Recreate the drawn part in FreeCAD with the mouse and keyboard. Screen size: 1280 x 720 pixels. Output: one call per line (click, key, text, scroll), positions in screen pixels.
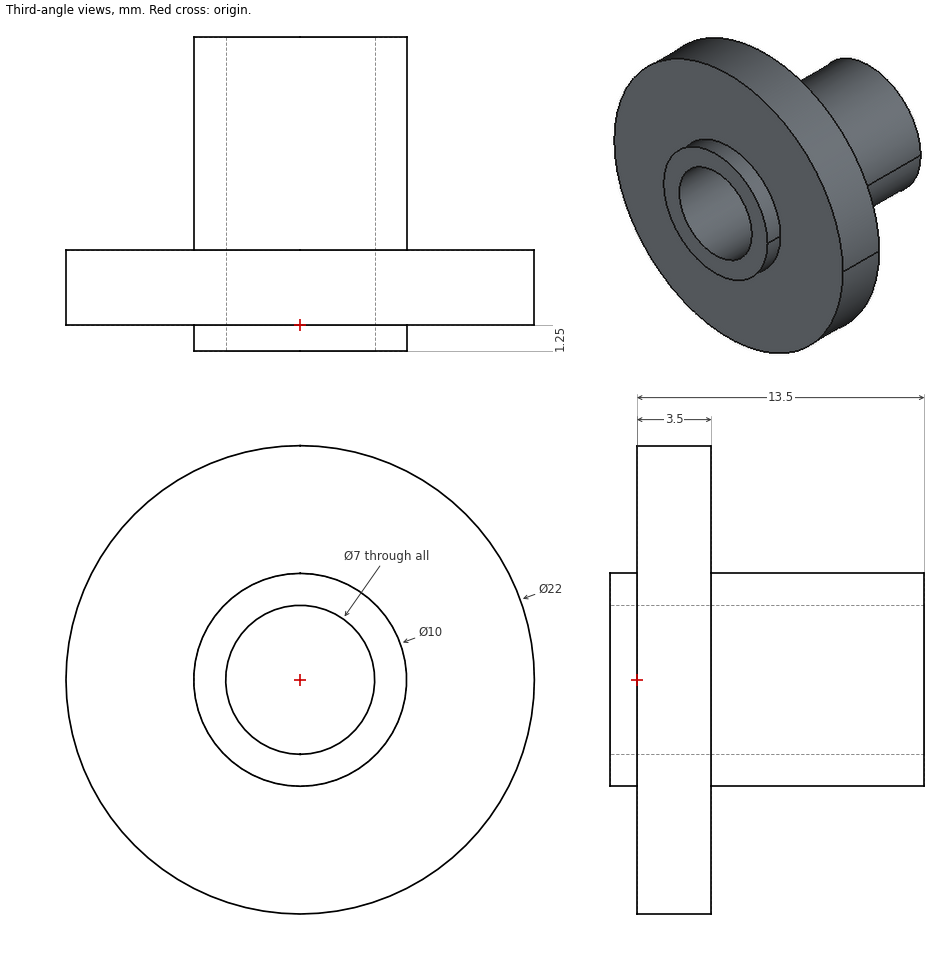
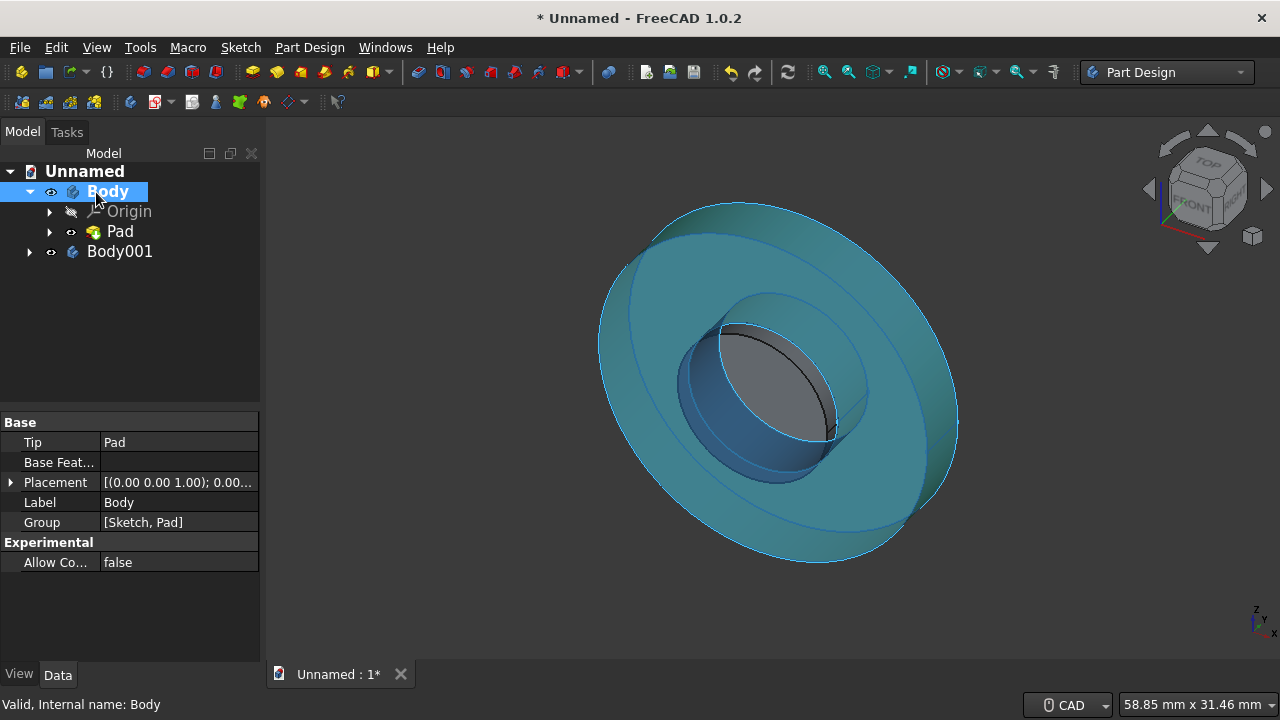
click(146, 562)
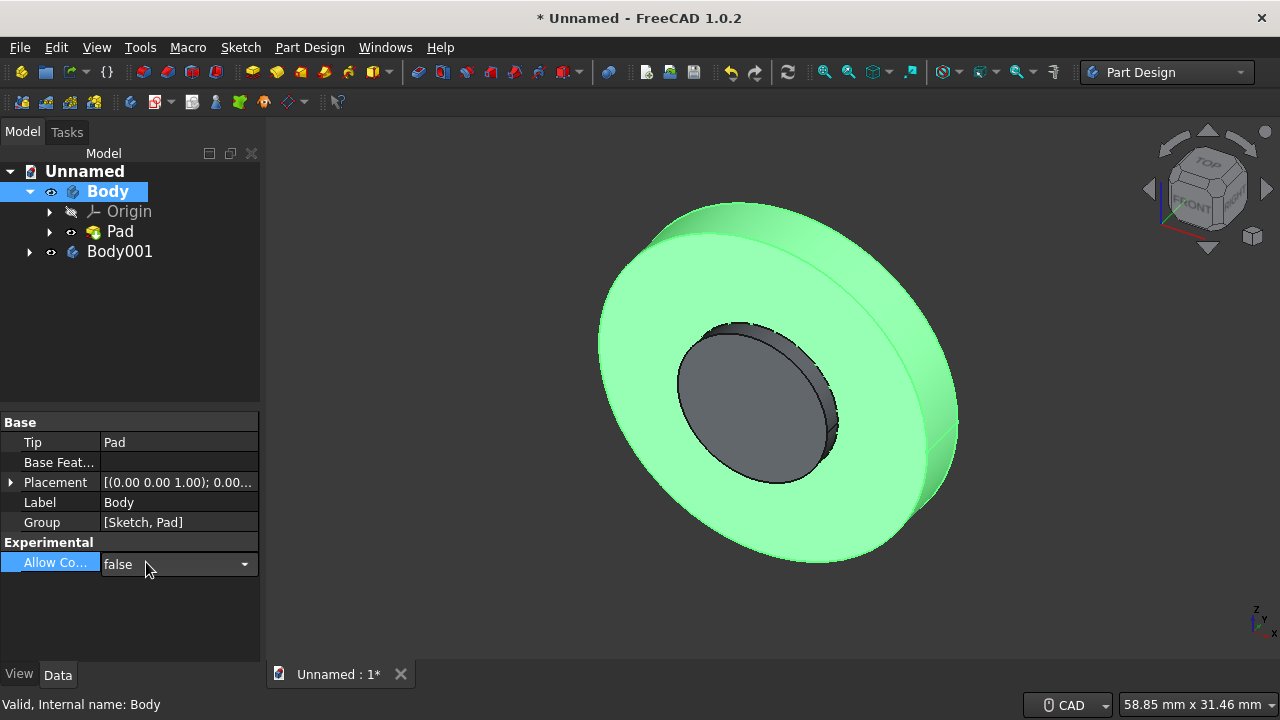
click(146, 562)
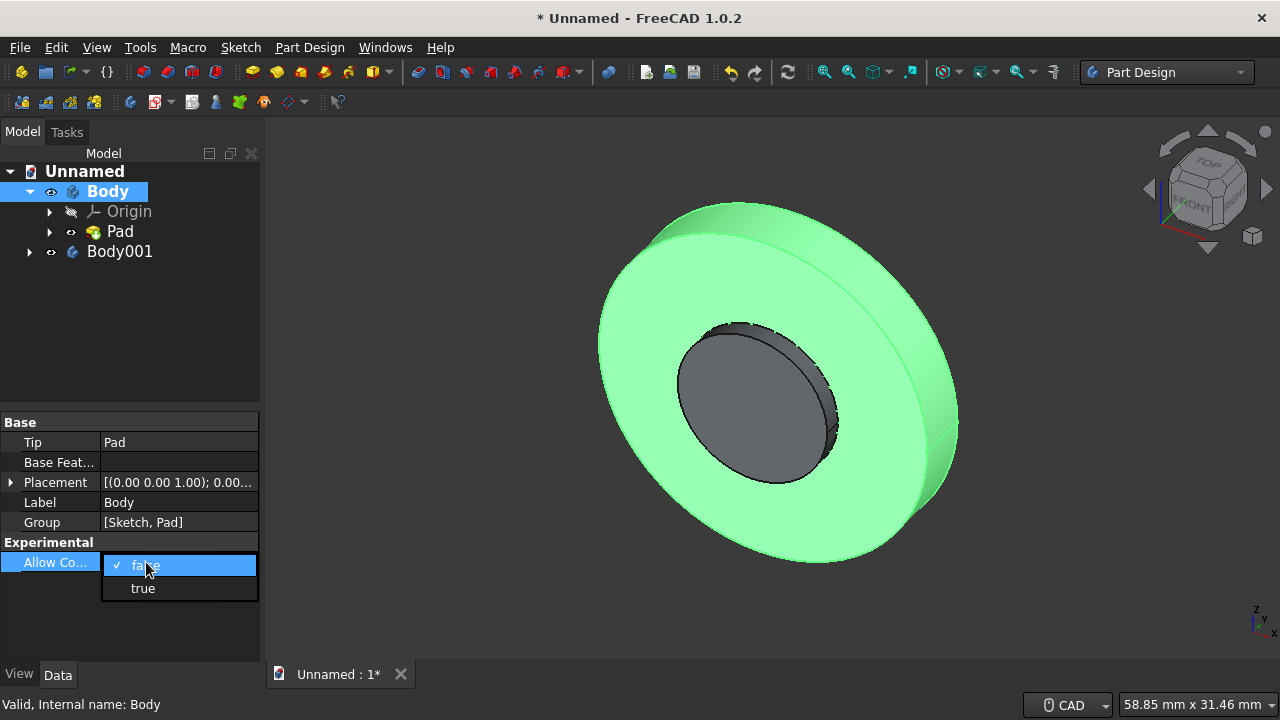
click(179, 588)
key(Return)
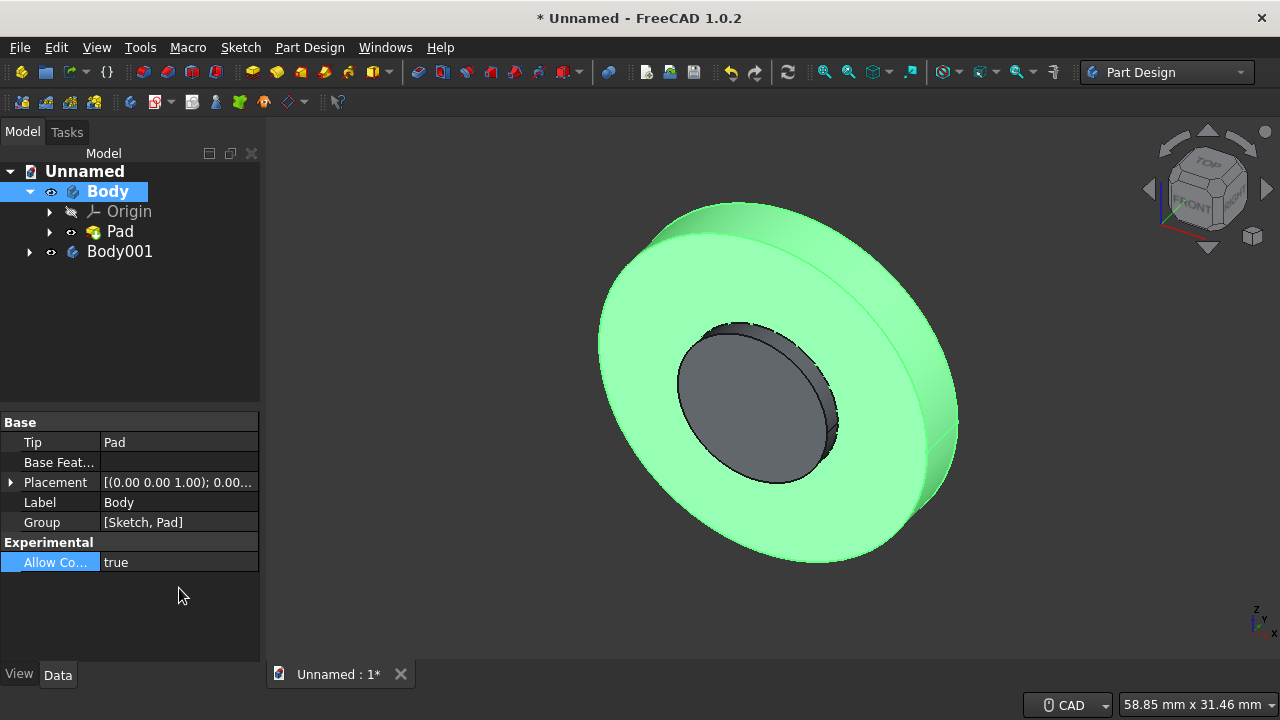
click(96, 252)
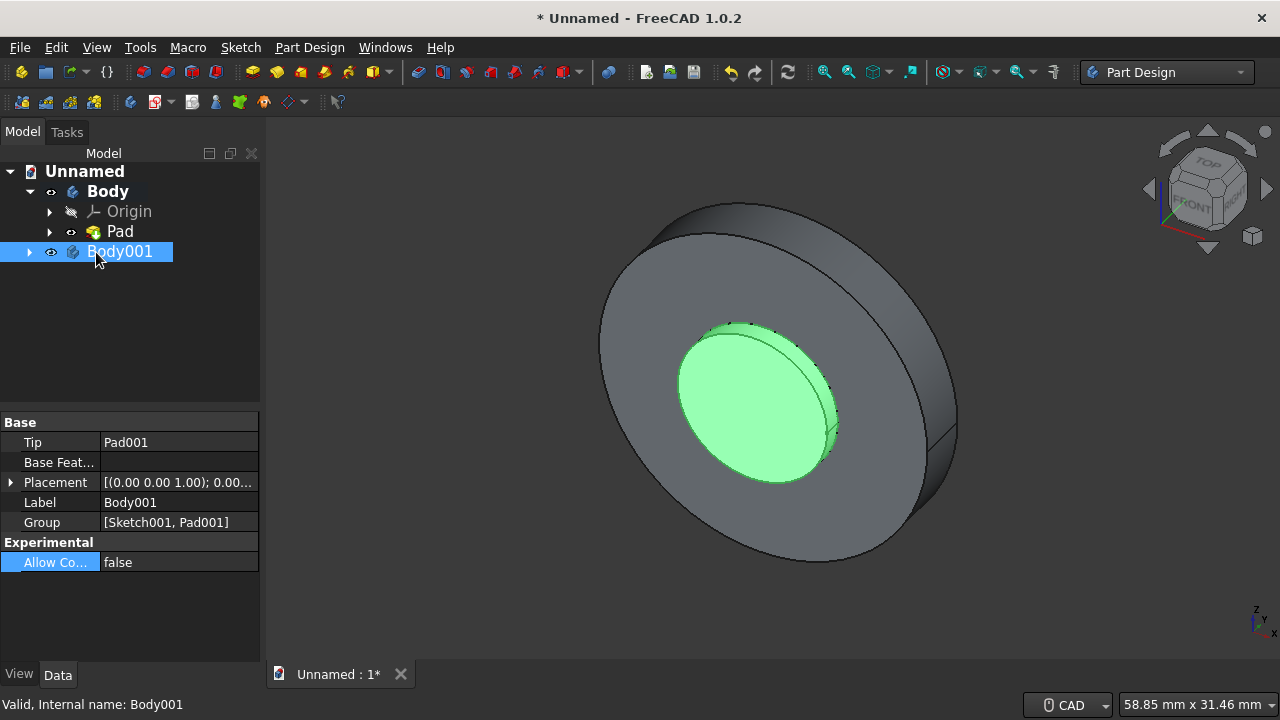
click(610, 72)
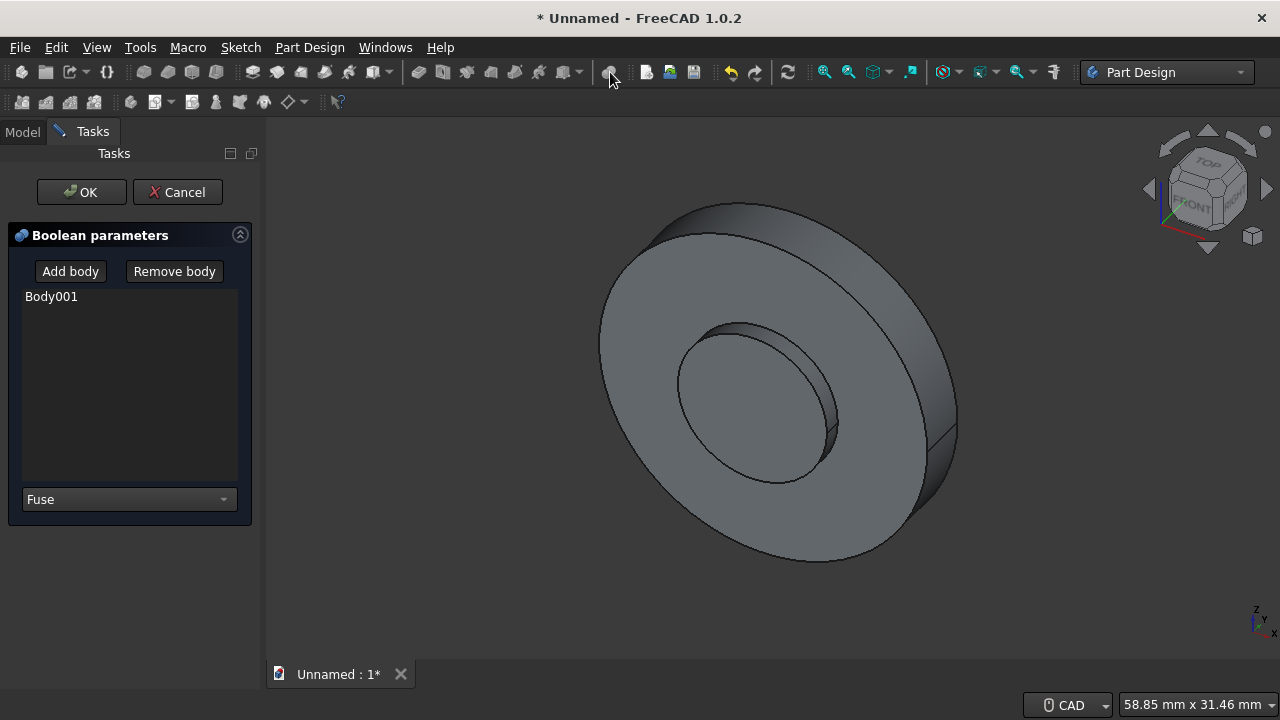
click(82, 192)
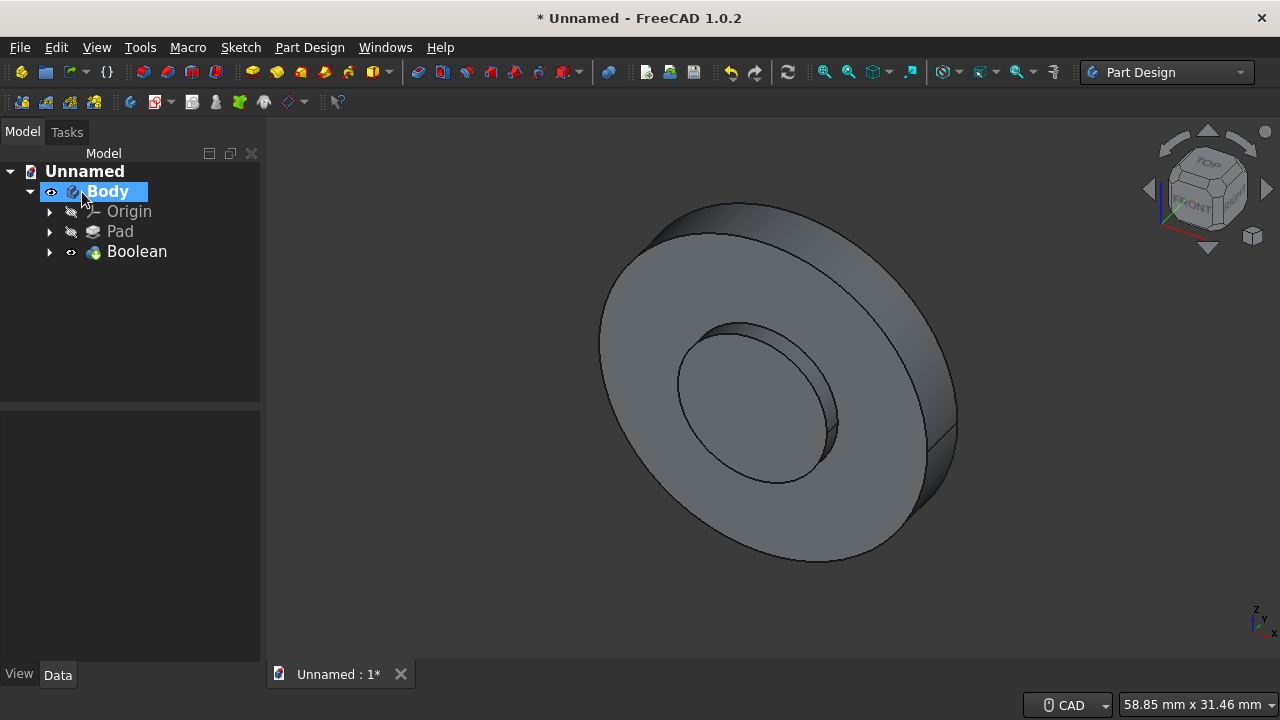
click(156, 102)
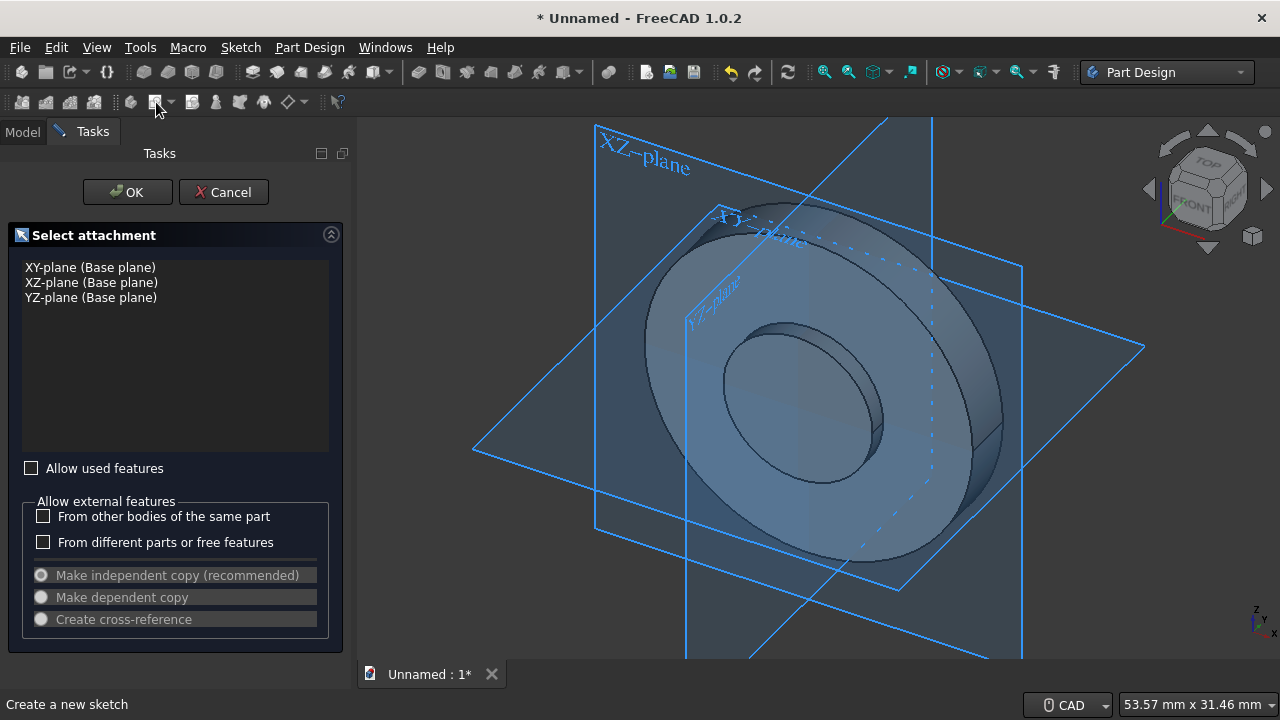
click(82, 282)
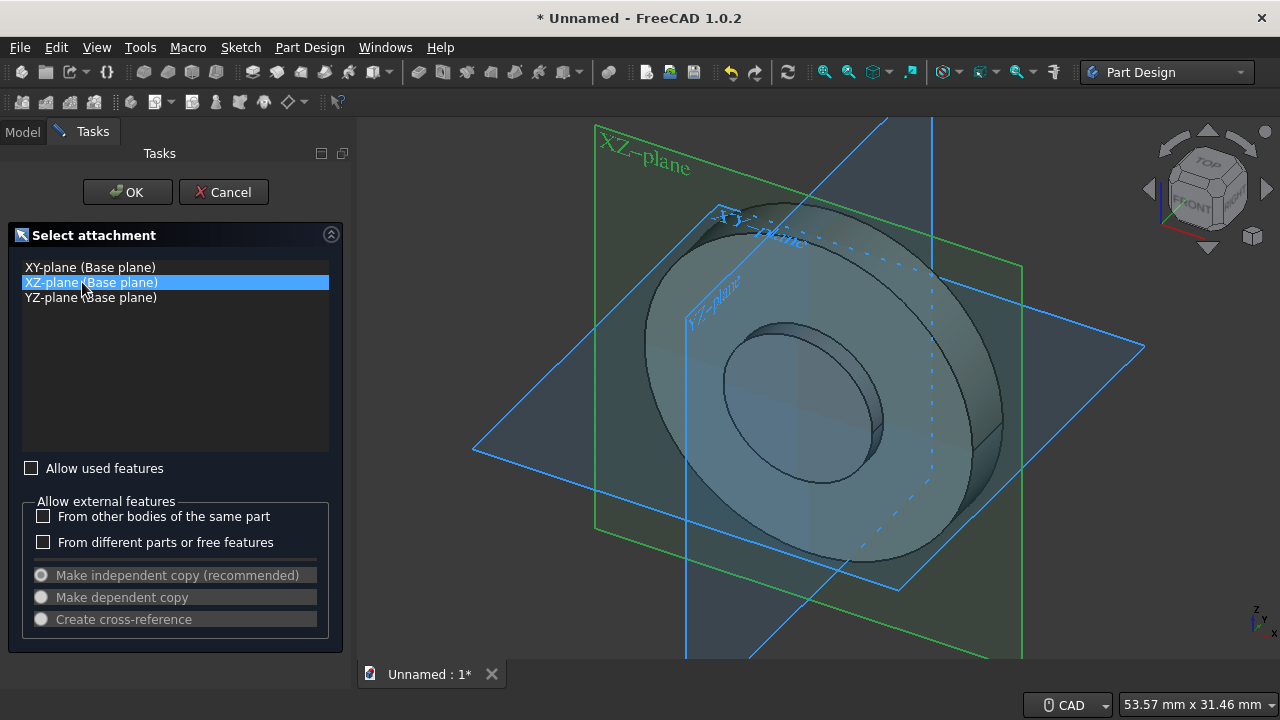
click(128, 192)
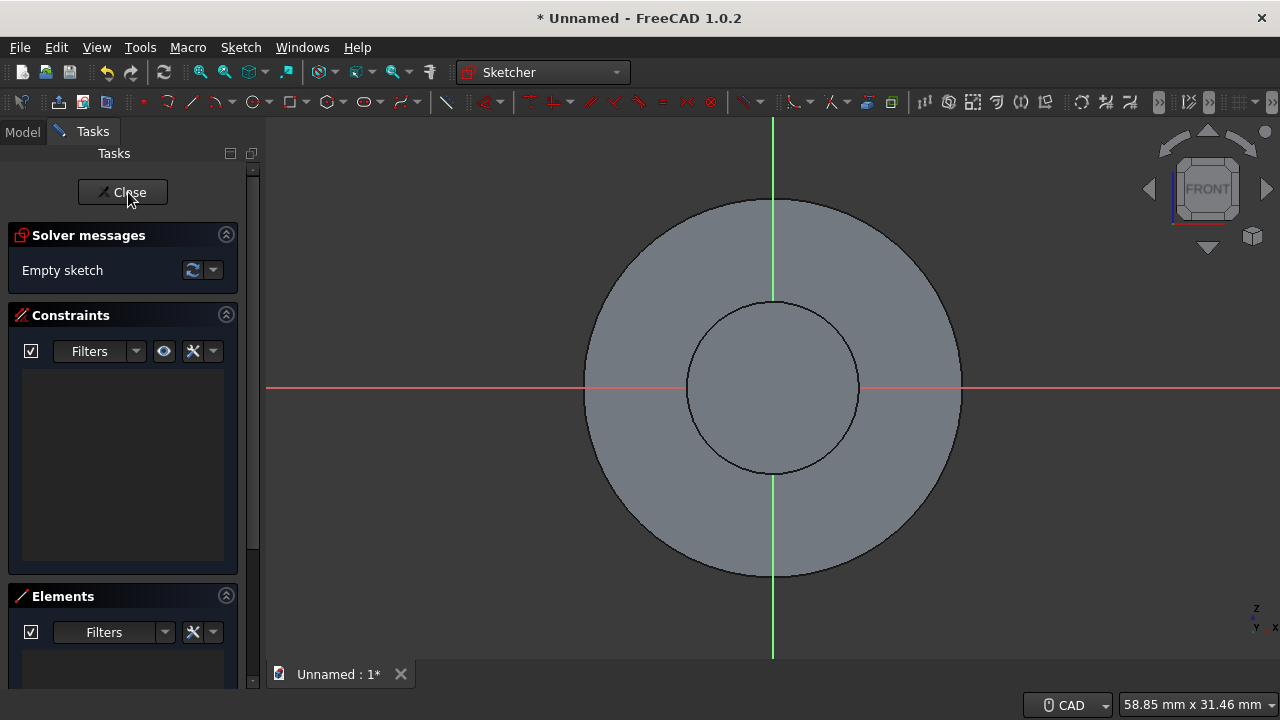
key(q)
key(s)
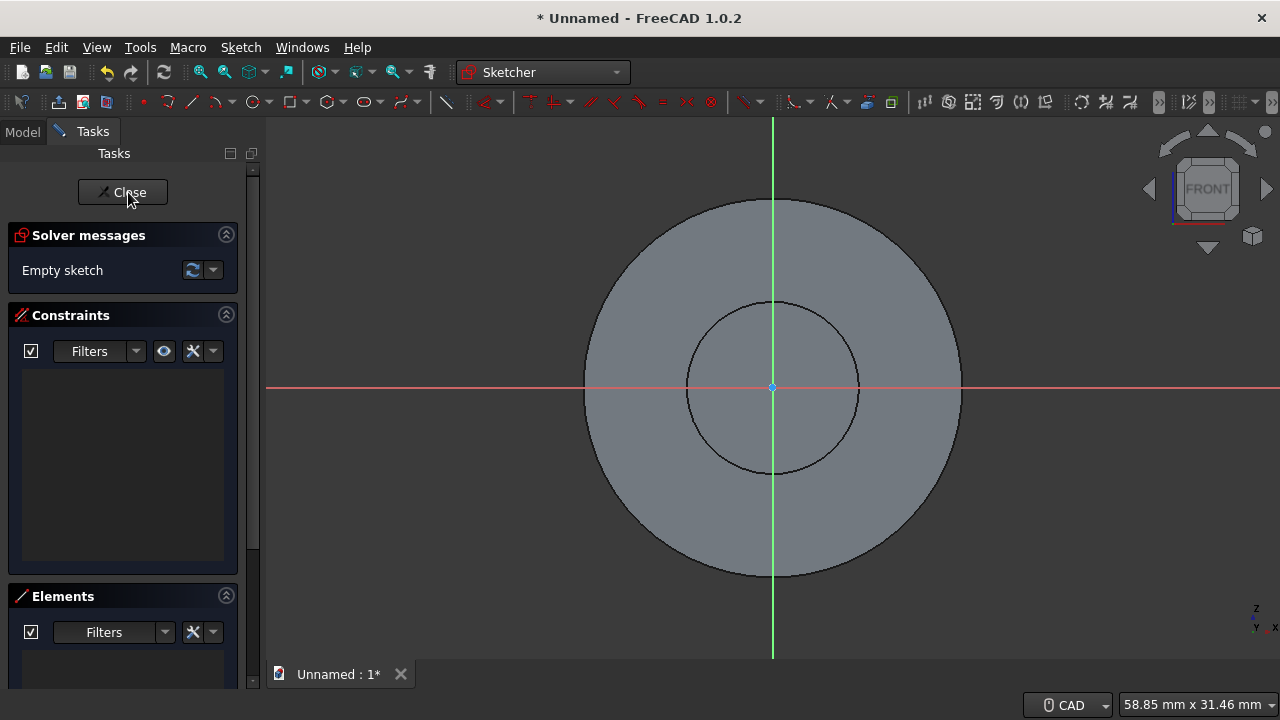
scroll(856, 388, up, 3)